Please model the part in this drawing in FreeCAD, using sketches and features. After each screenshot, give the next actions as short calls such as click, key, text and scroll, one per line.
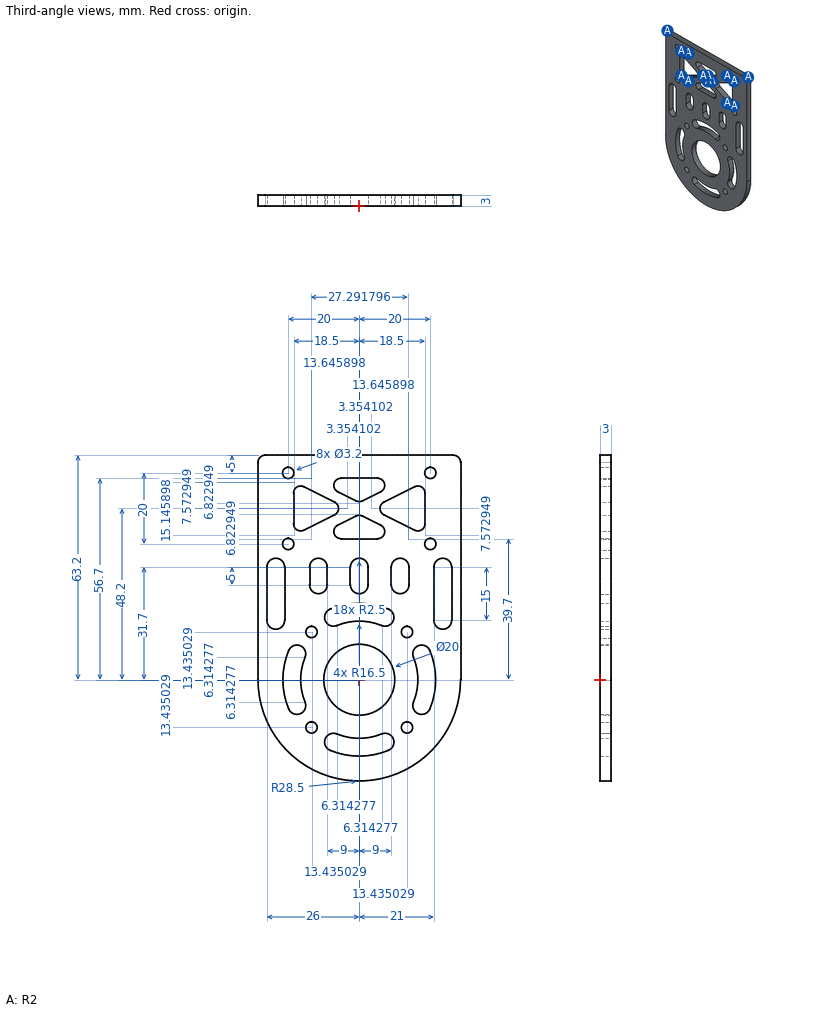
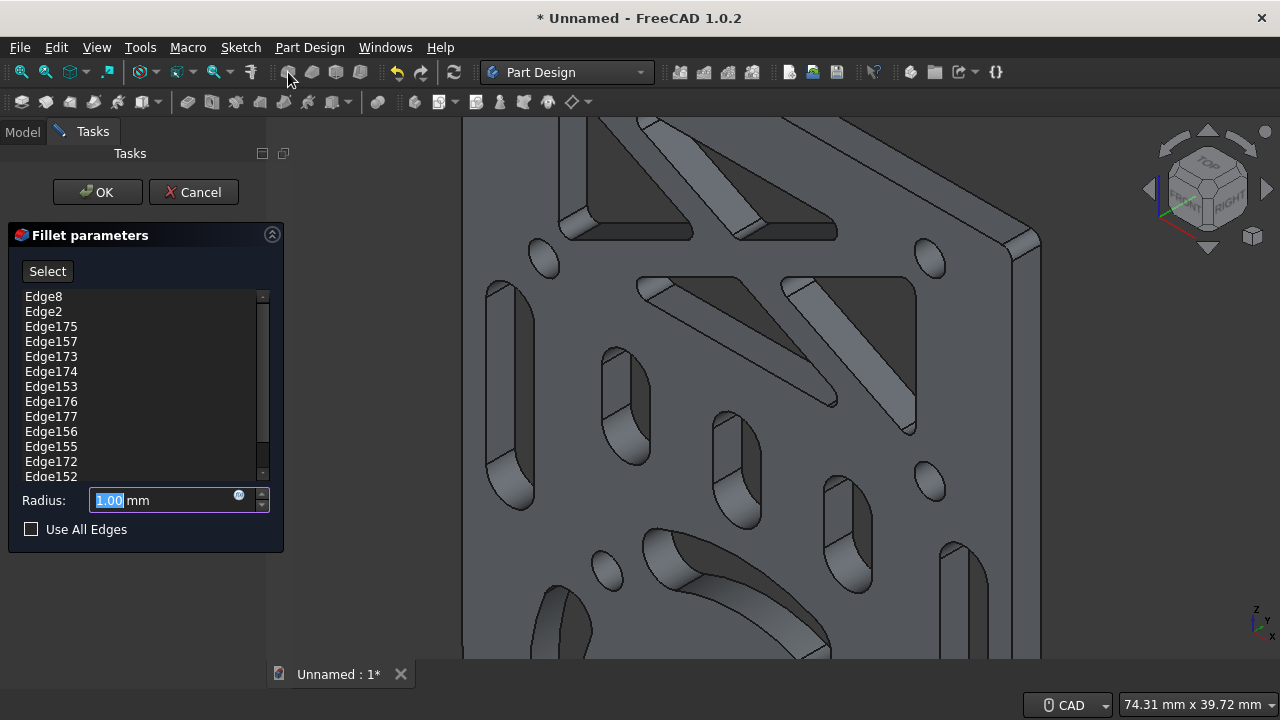
text(2)
key(Tab)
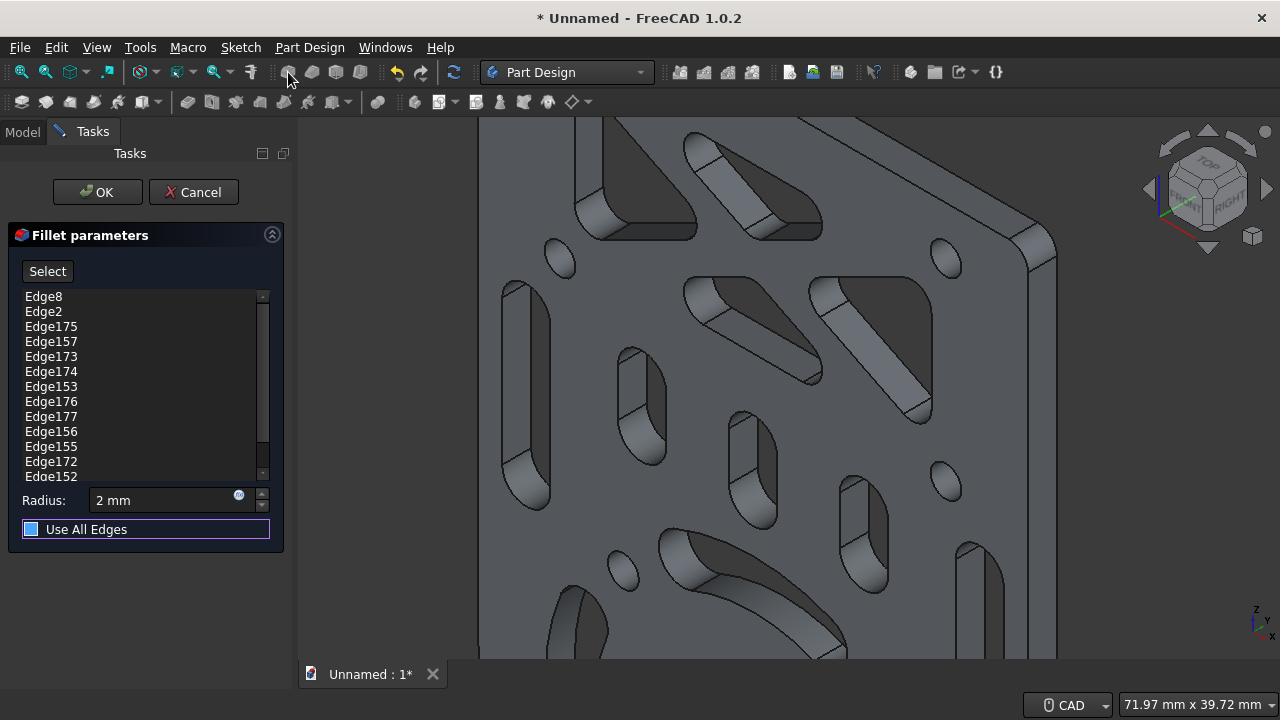
click(98, 192)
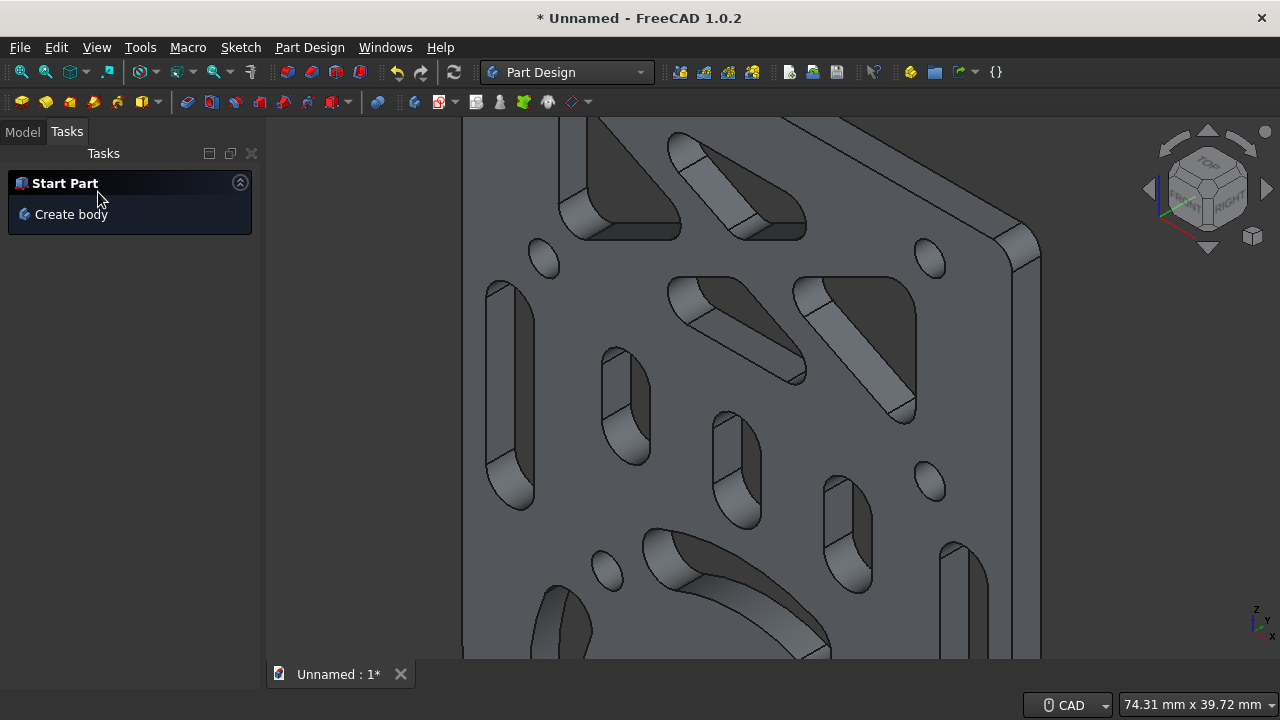
key(v)
key(f)